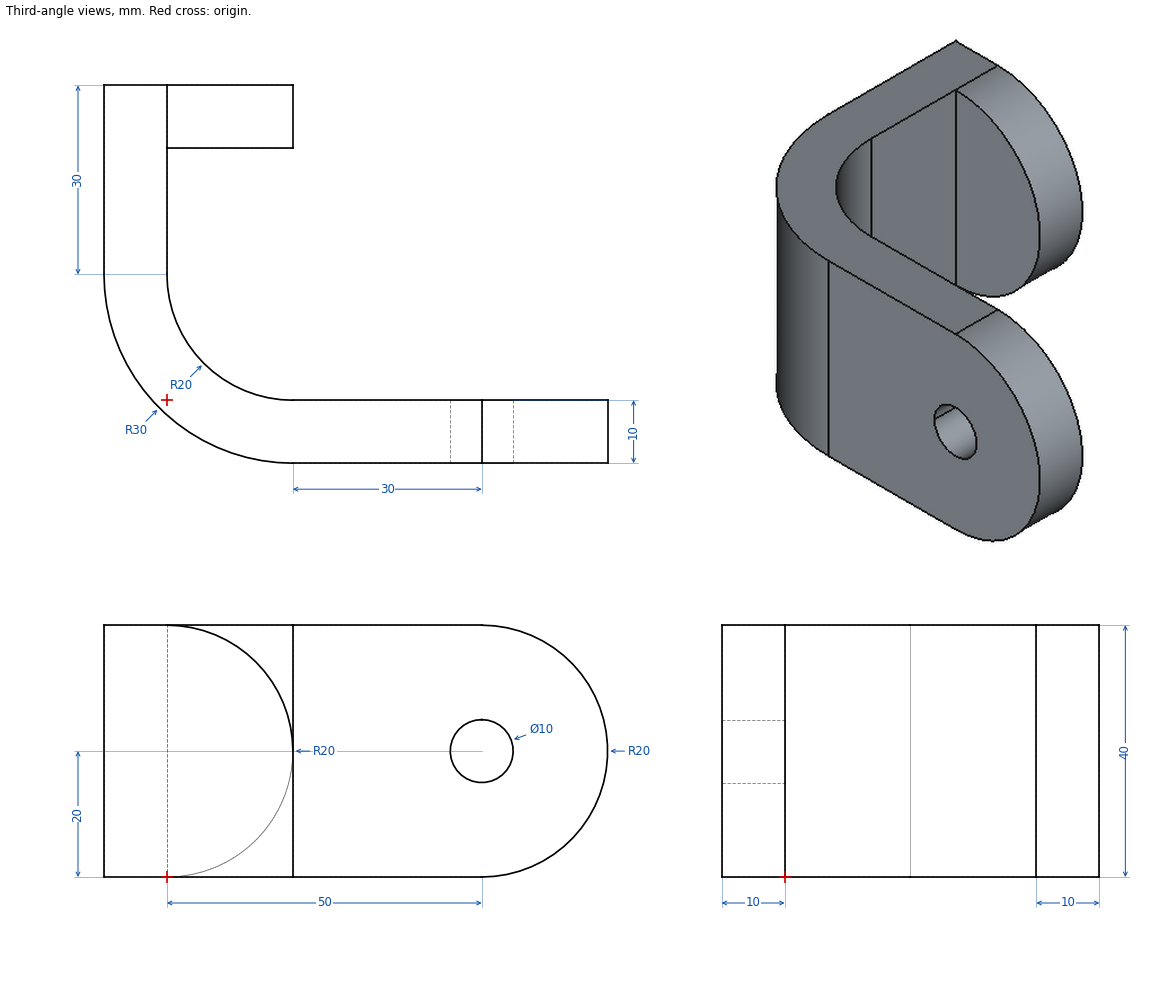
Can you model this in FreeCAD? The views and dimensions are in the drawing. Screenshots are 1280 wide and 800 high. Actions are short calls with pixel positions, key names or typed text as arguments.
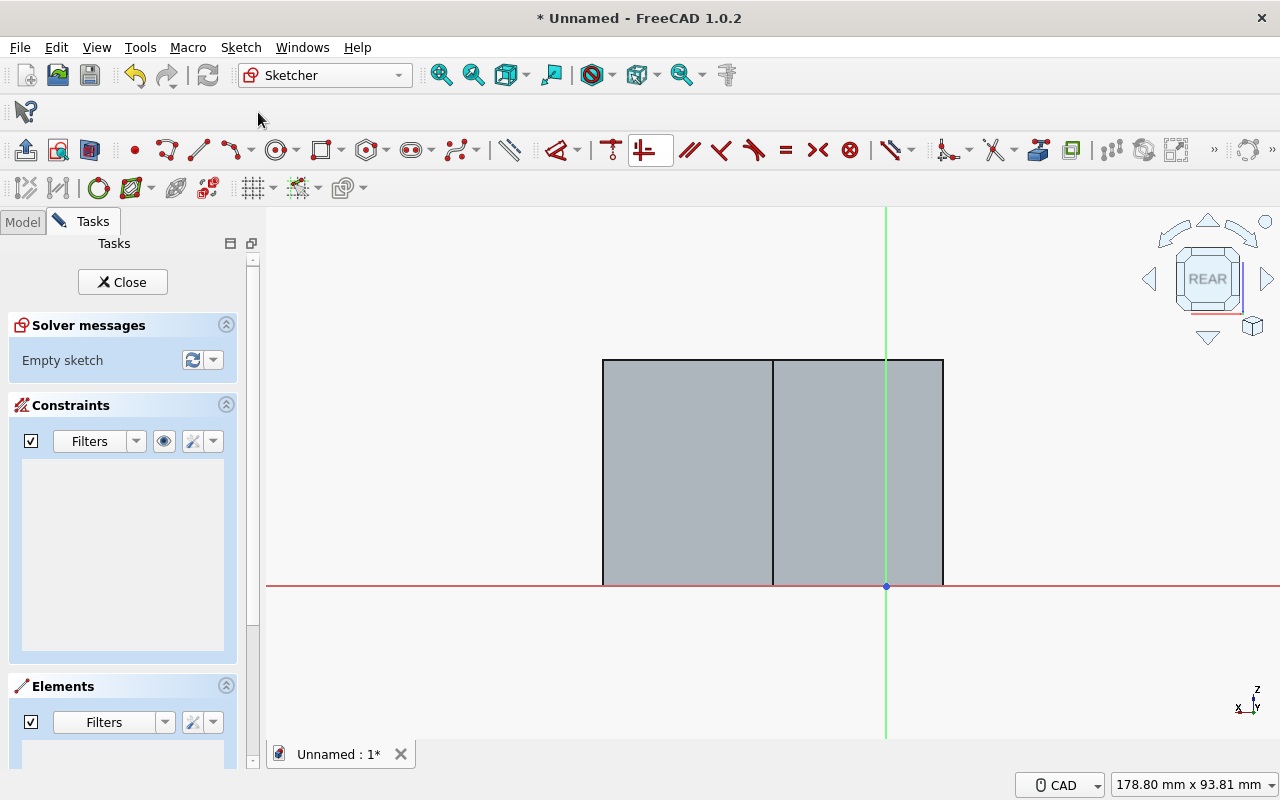
scroll(1084, 473, up, 2)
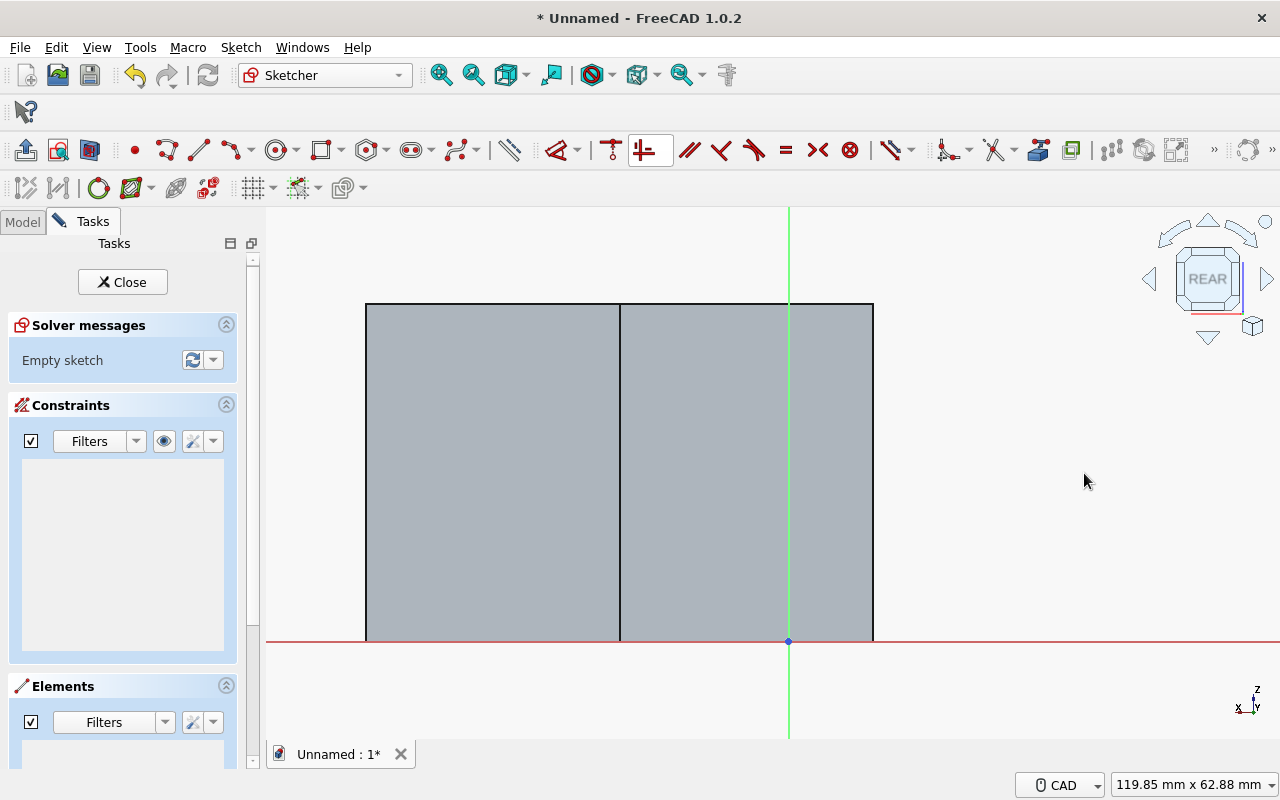
key(g)
key(l)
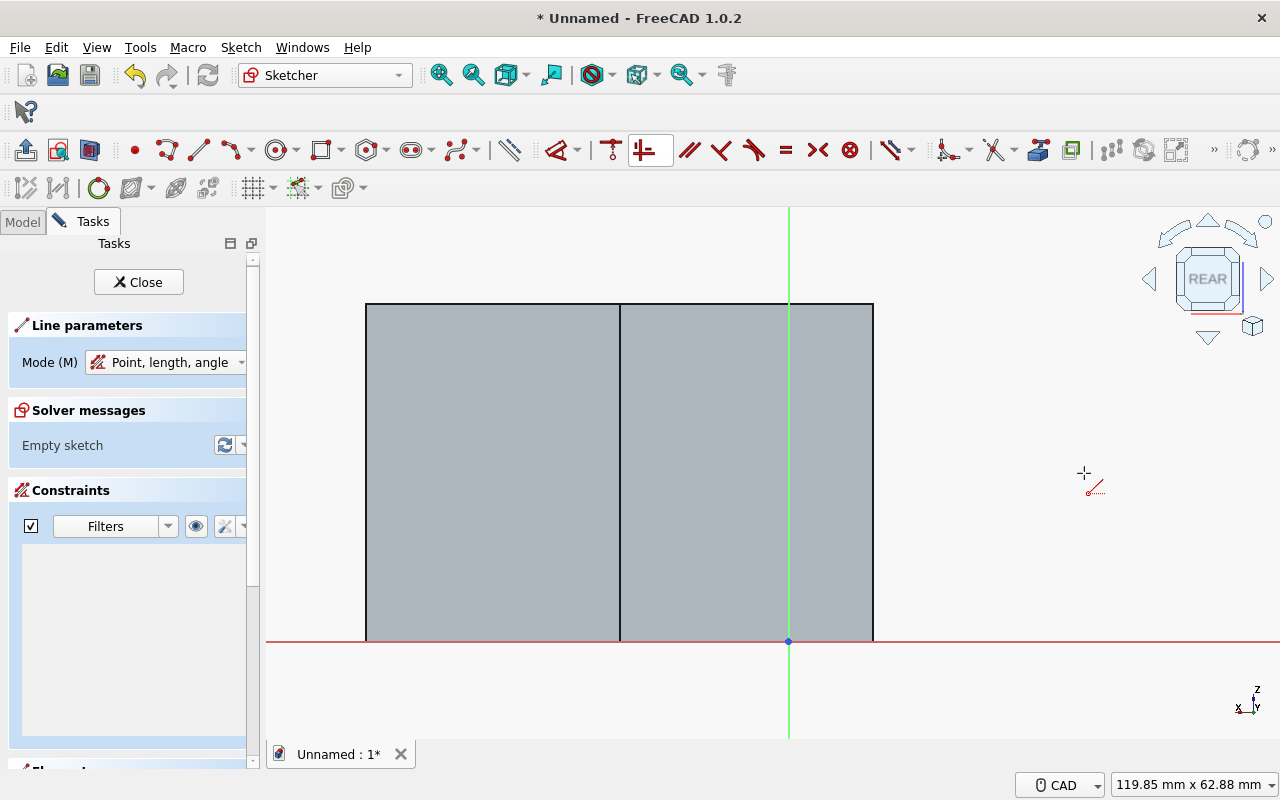
click(789, 642)
click(780, 304)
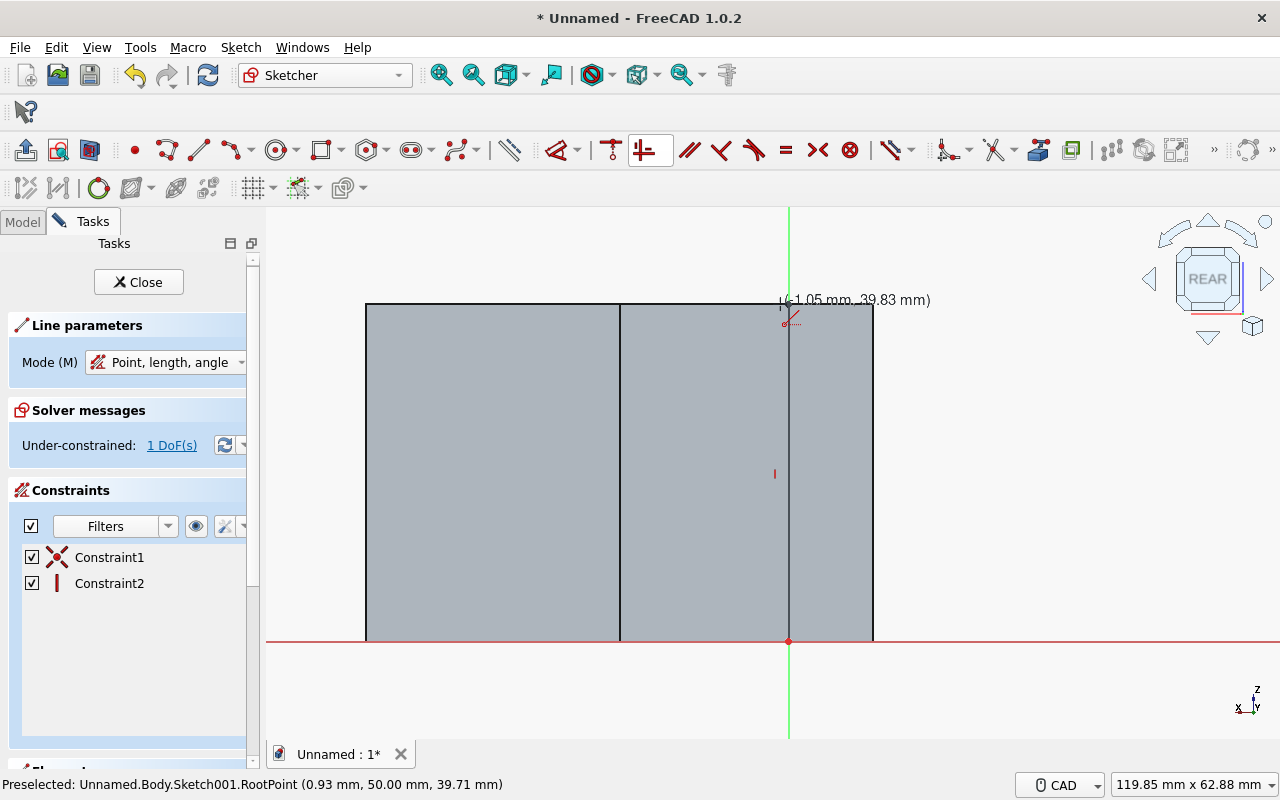
click(232, 150)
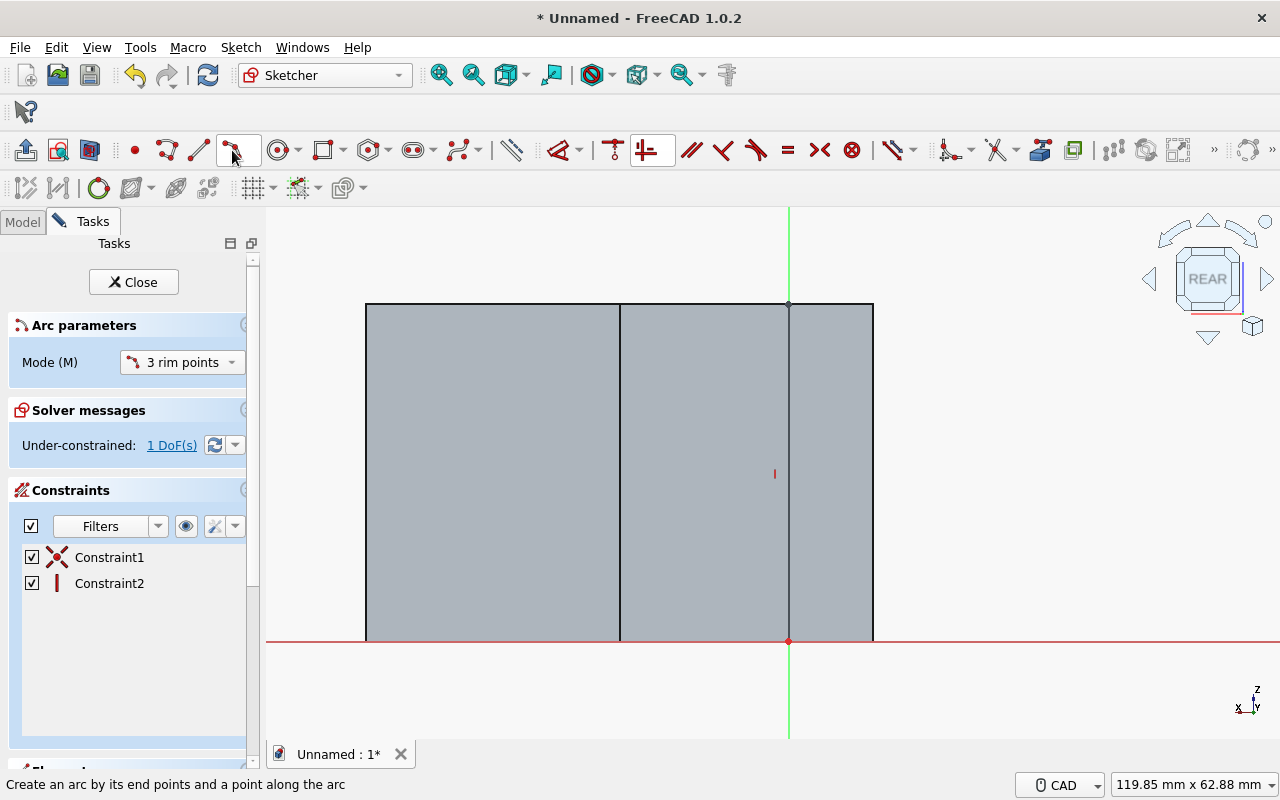
click(789, 305)
click(789, 642)
click(620, 473)
key(Escape)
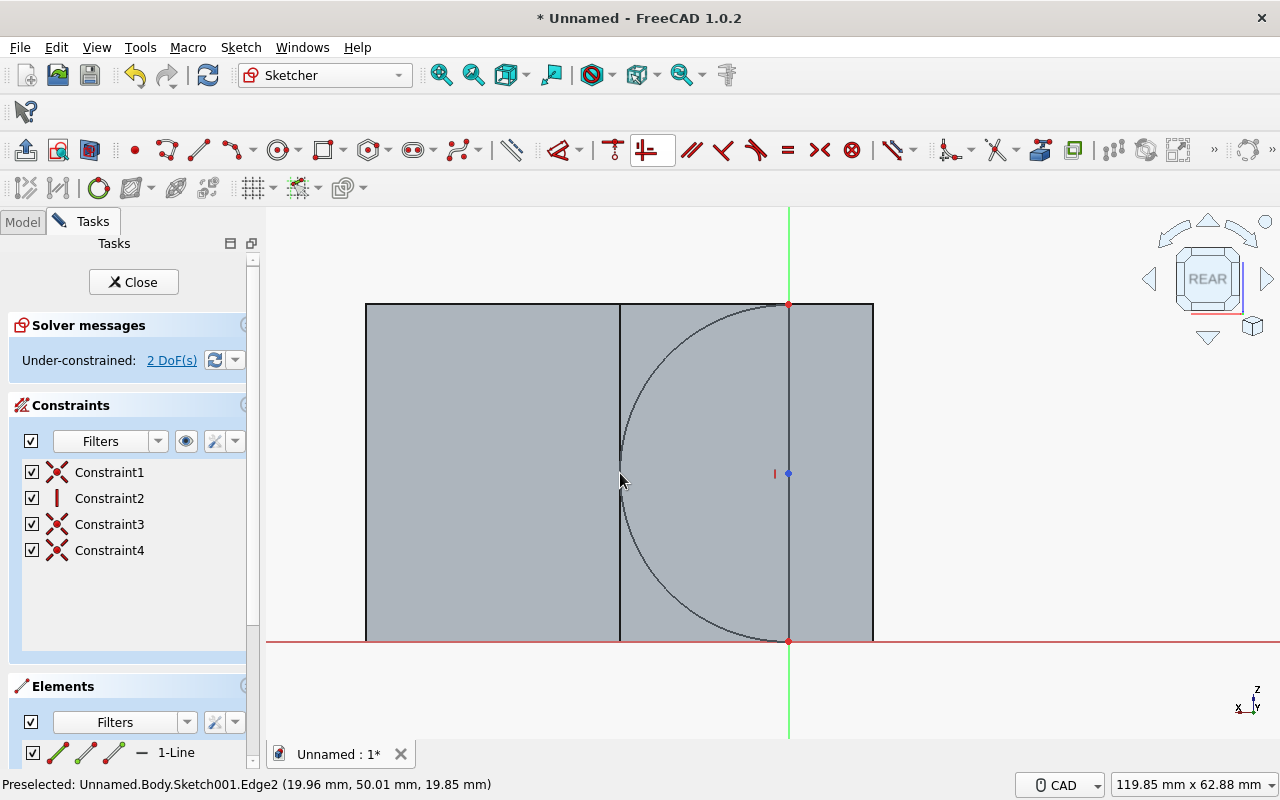
click(788, 473)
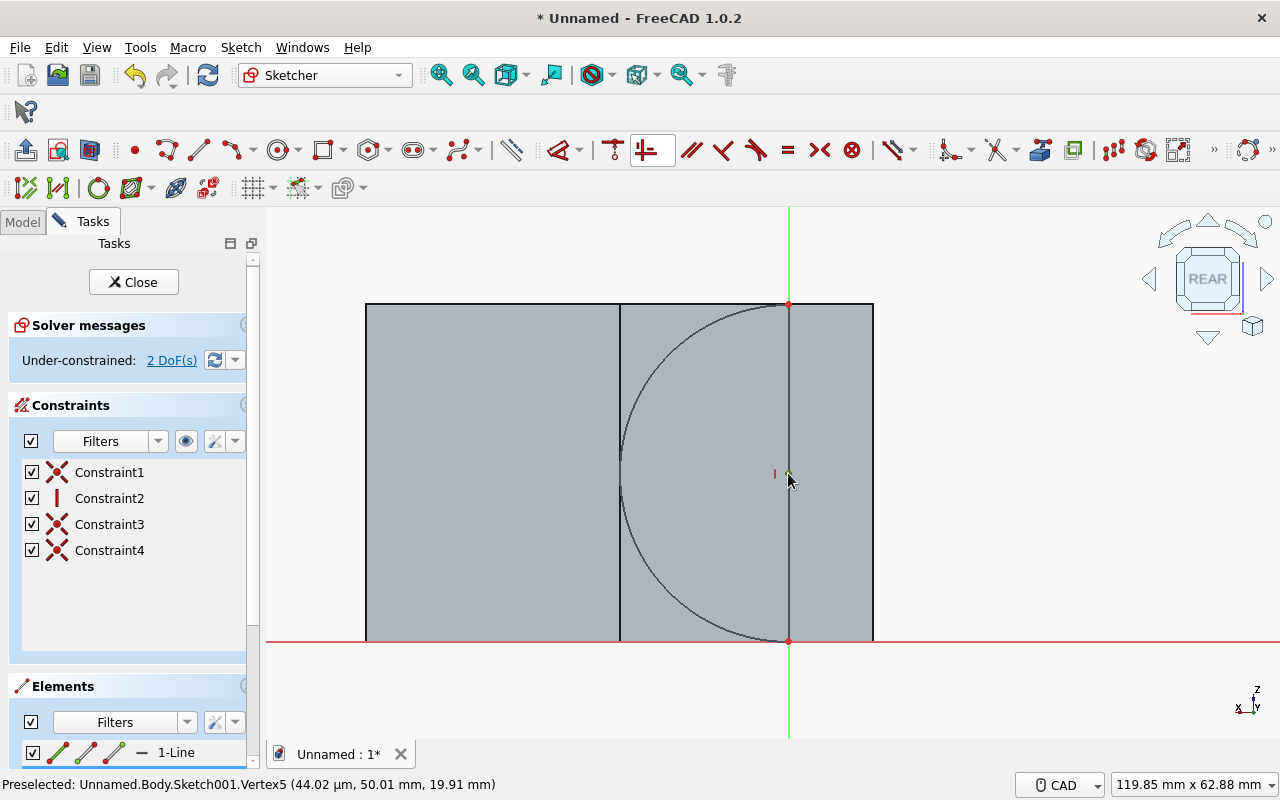
click(789, 677)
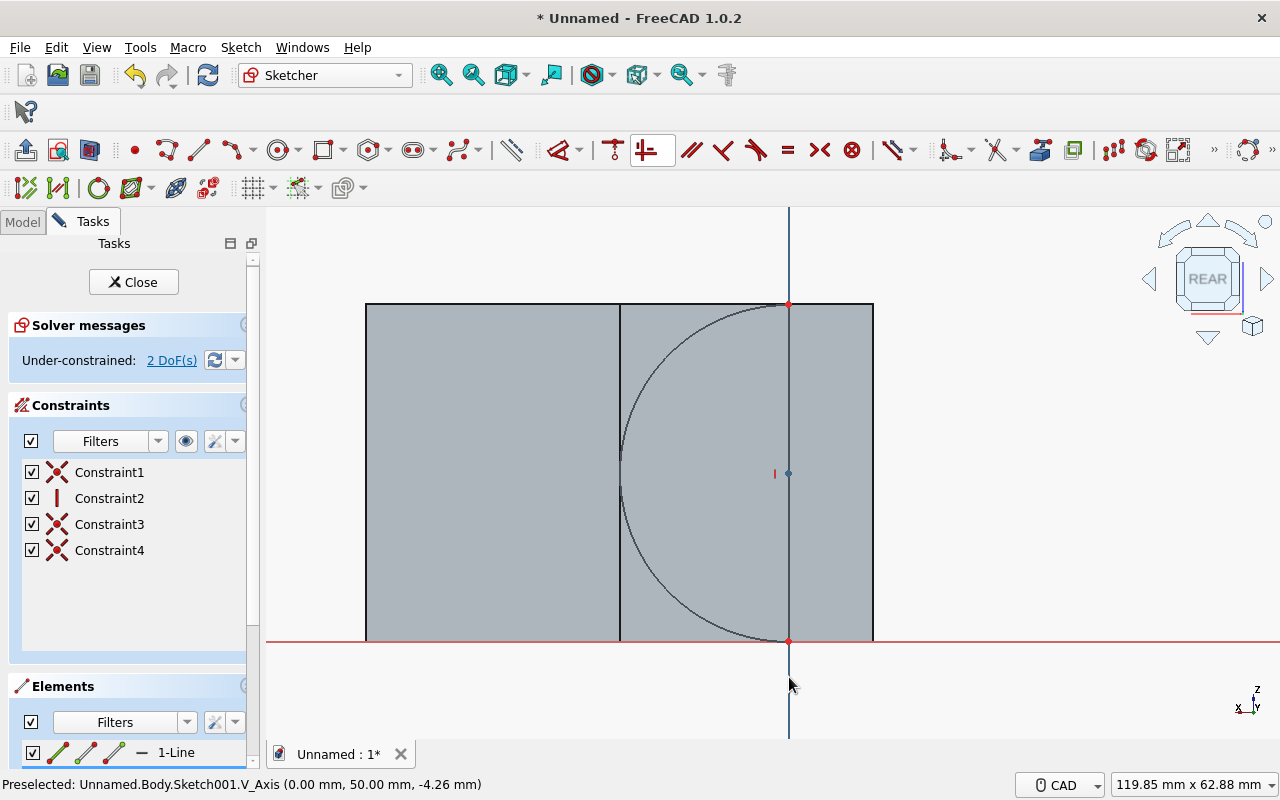
key(c)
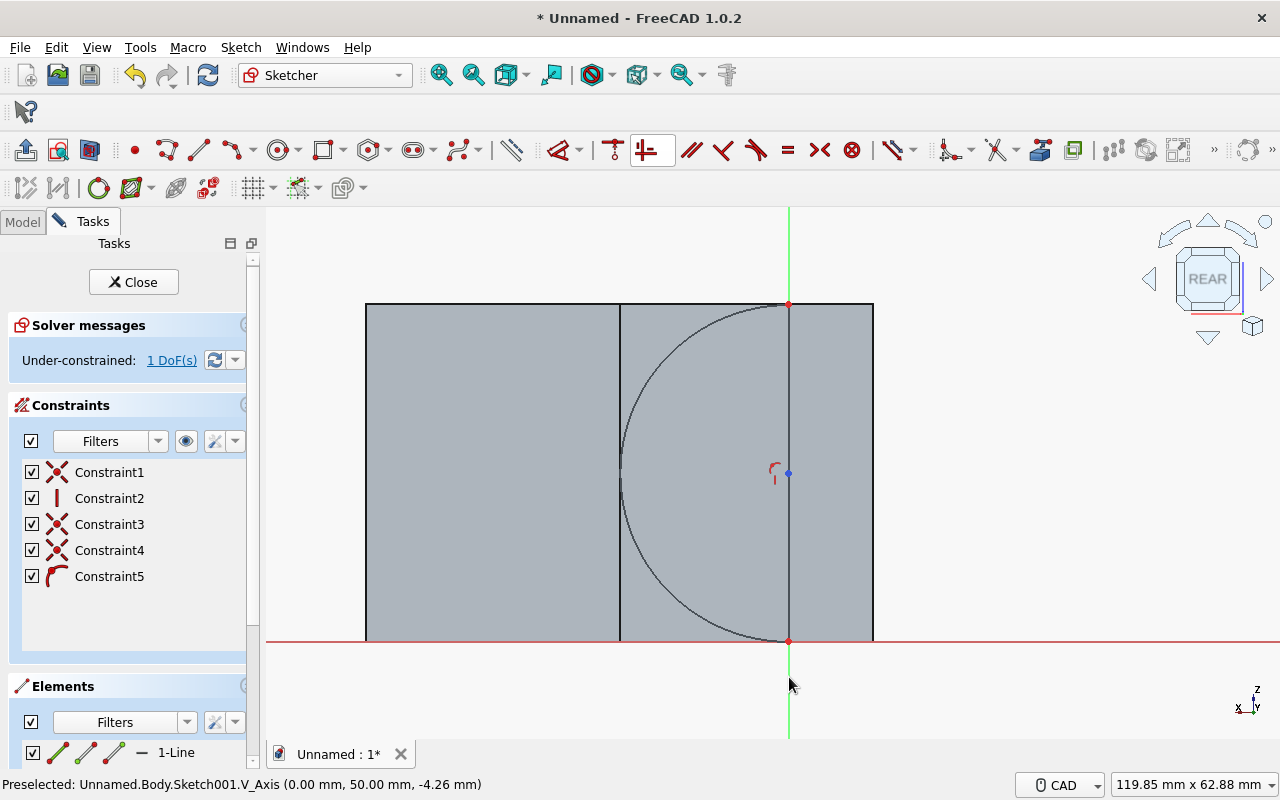
key(d)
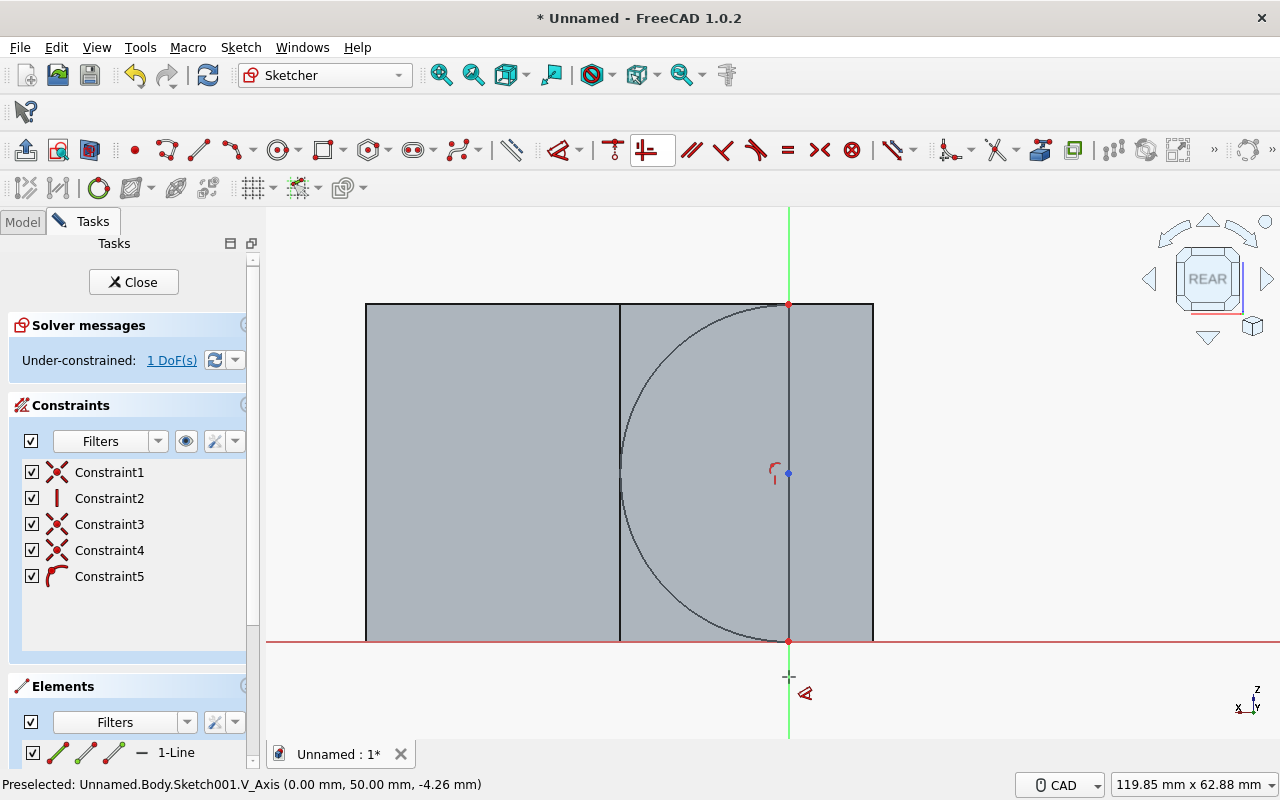
click(653, 374)
click(627, 355)